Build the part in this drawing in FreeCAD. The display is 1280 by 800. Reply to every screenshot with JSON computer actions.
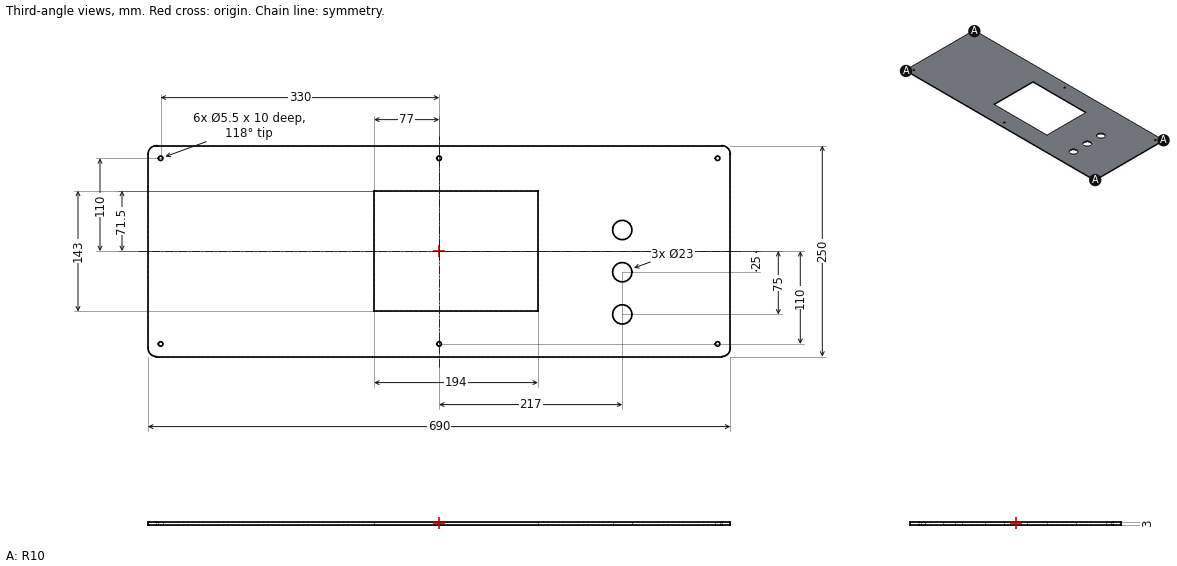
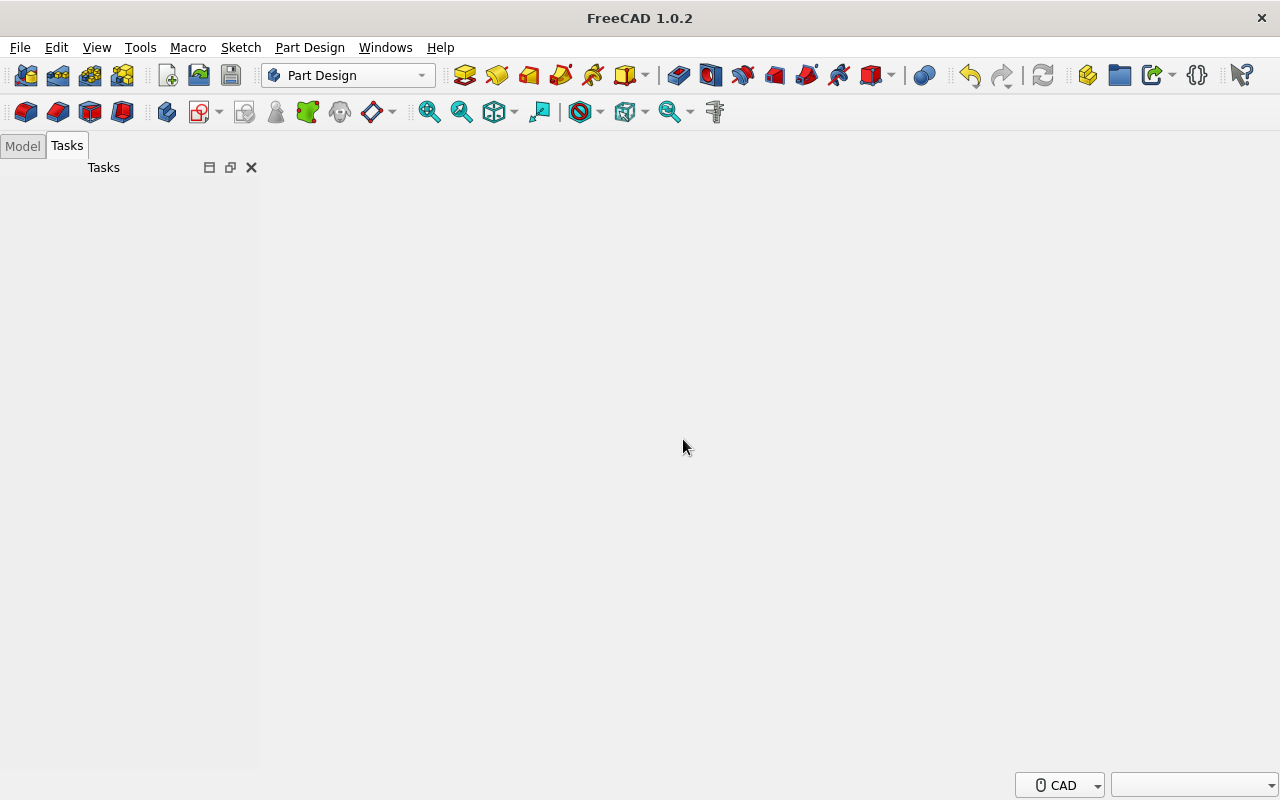
{"action": "left_click", "coordinate": [168, 76]}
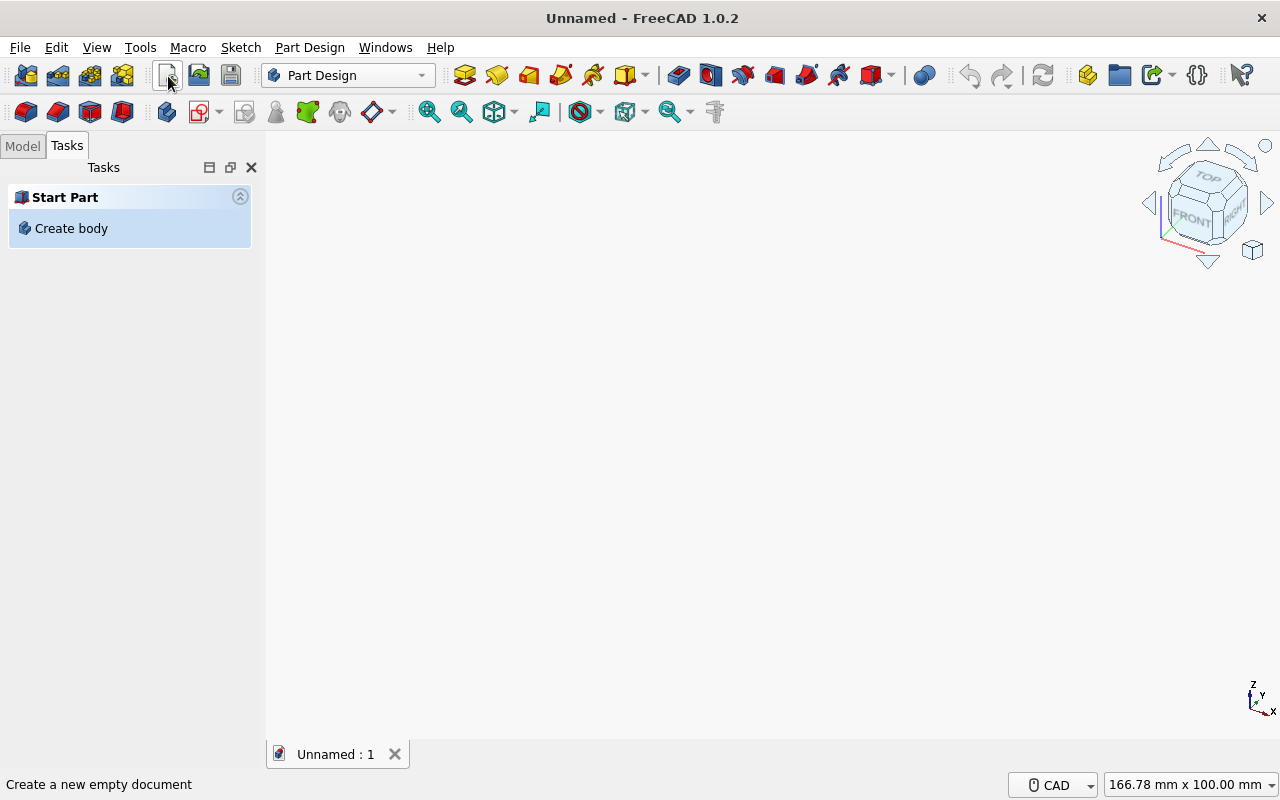
{"action": "left_click", "coordinate": [200, 112]}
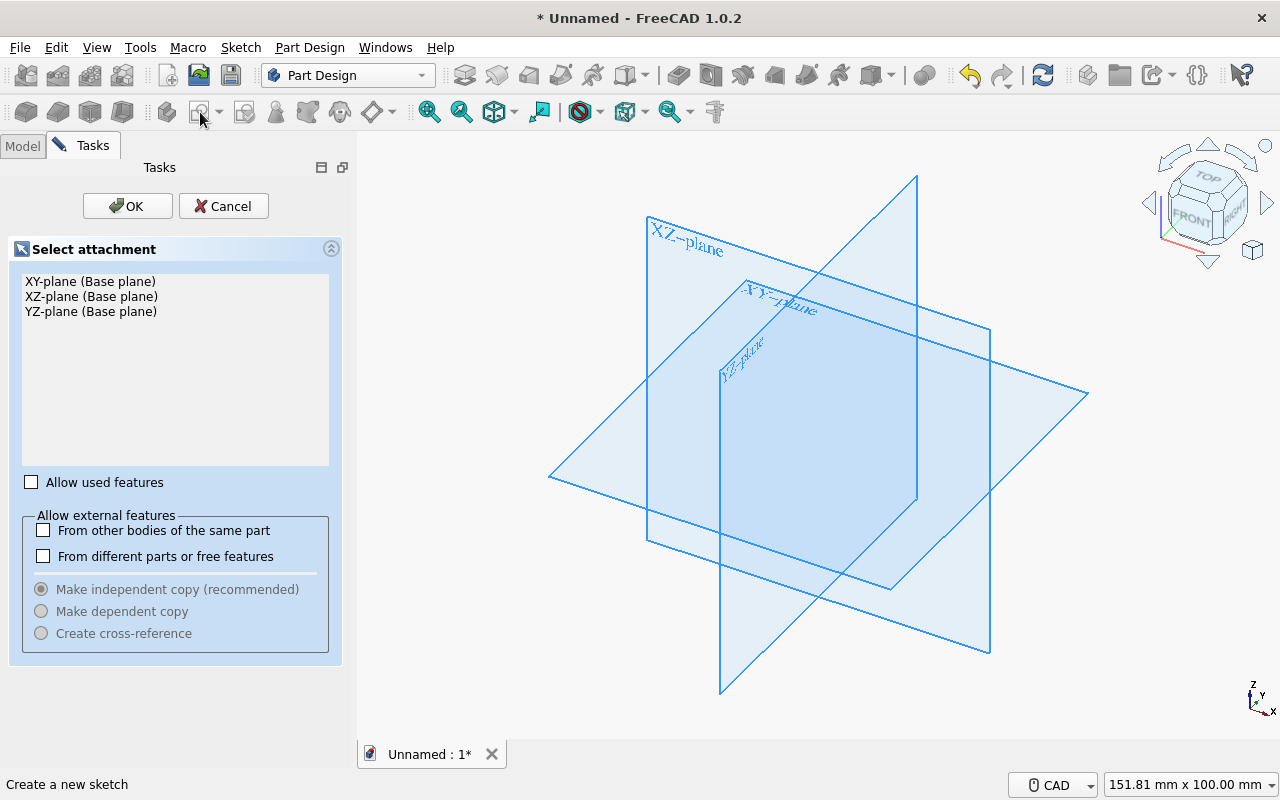
{"action": "left_click", "coordinate": [82, 282]}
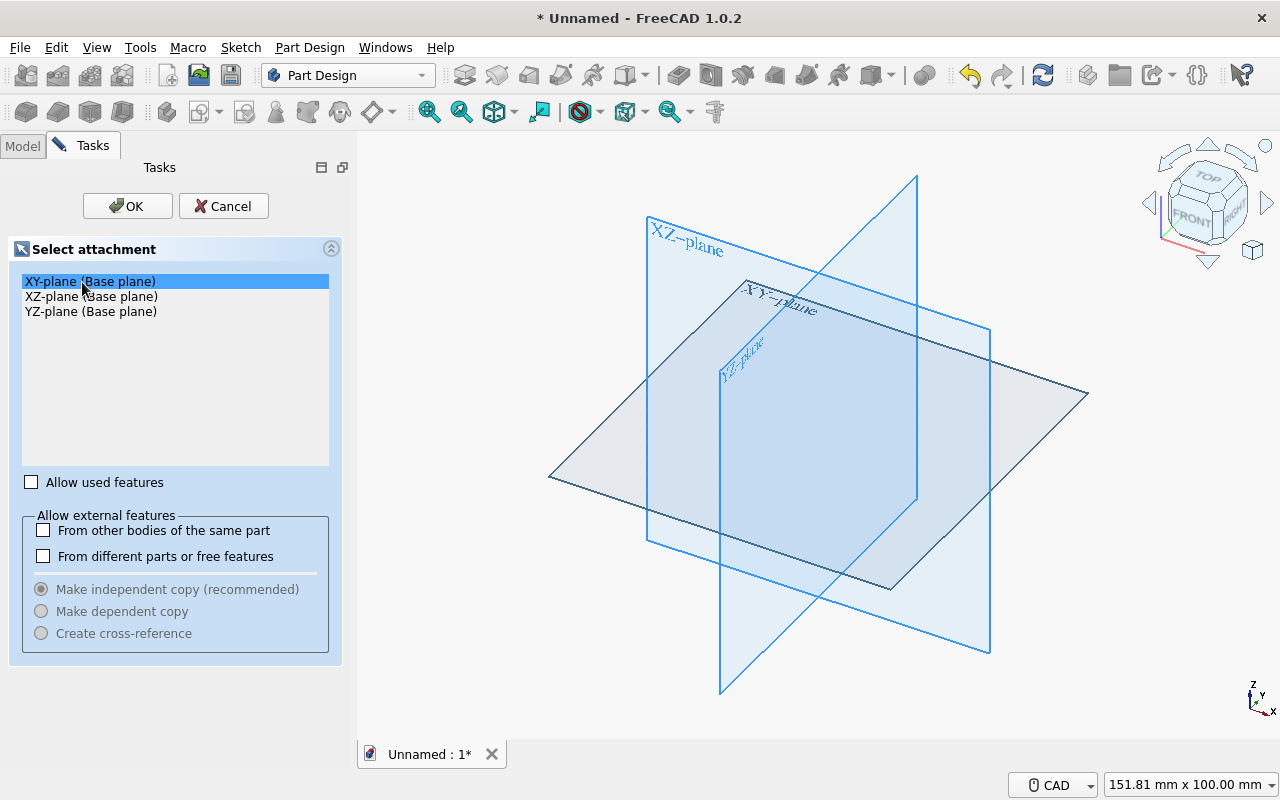
{"action": "left_click", "coordinate": [128, 206]}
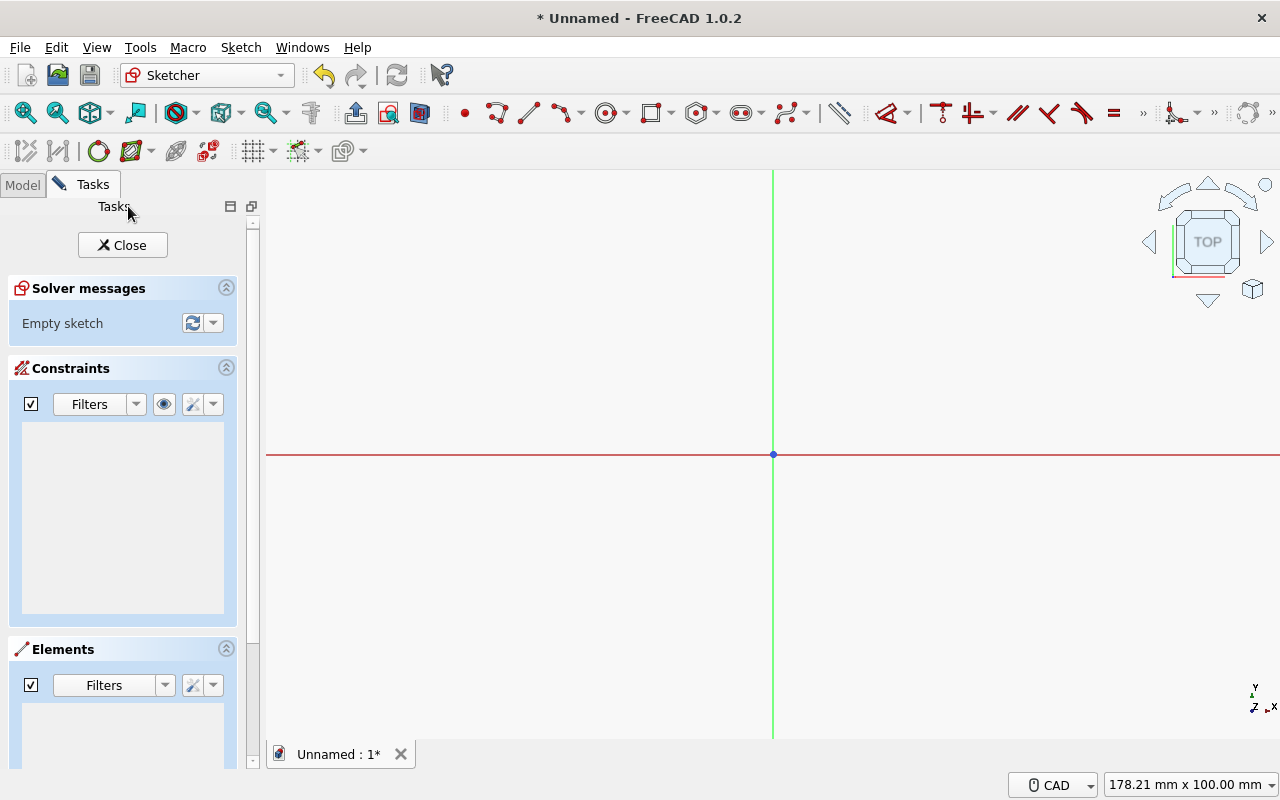
{"action": "scroll", "coordinate": [694, 454], "scroll_direction": "down", "scroll_amount": 10}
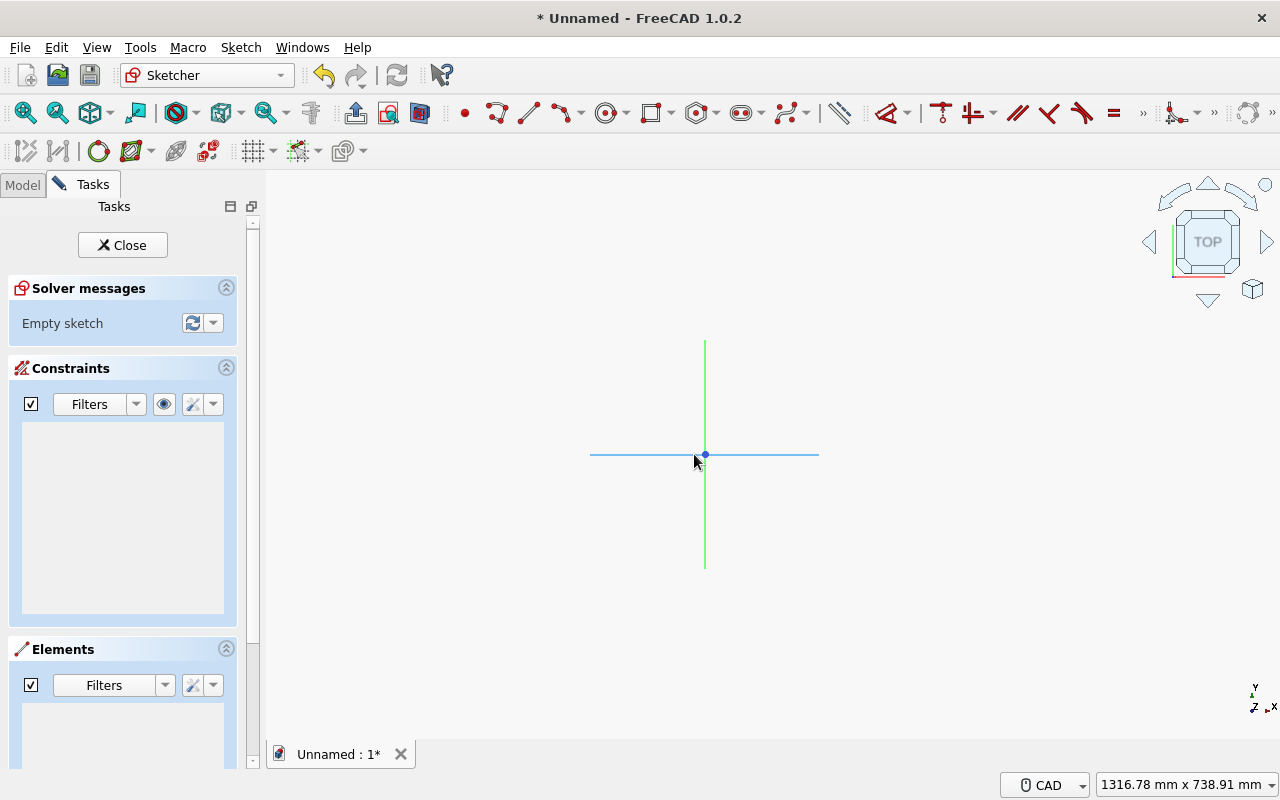
{"action": "key", "text": "g v"}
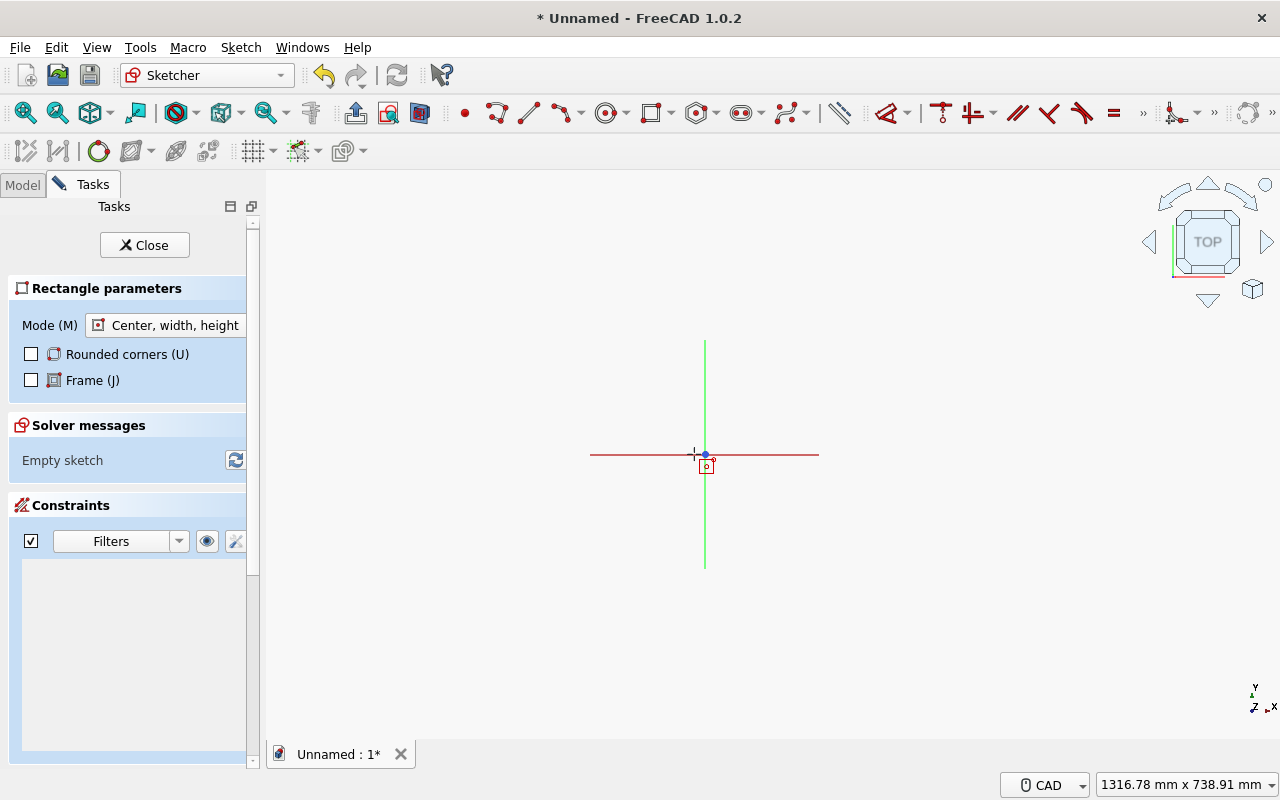
{"action": "left_click", "coordinate": [705, 454]}
{"action": "left_click", "coordinate": [971, 358]}
{"action": "key", "text": "Escape"}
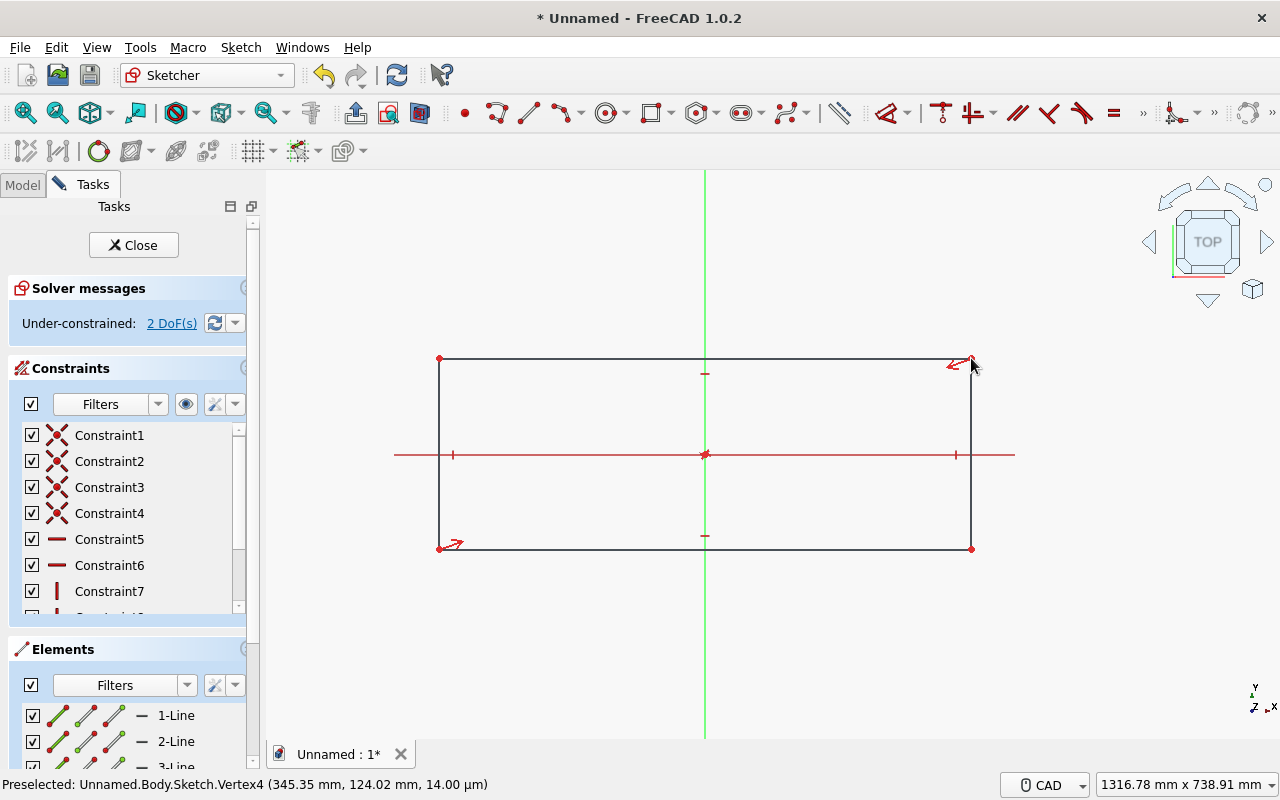
{"action": "left_click", "coordinate": [599, 550]}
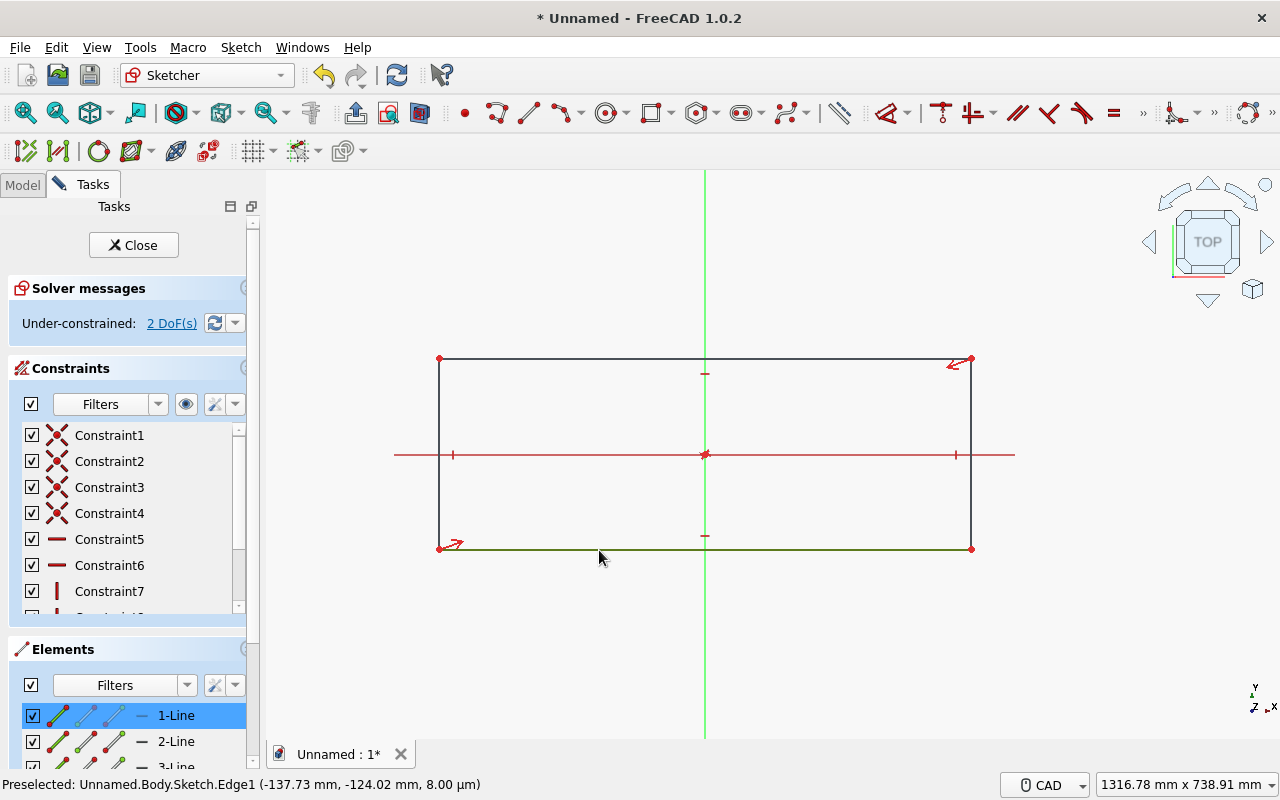
{"action": "left_click", "coordinate": [910, 114]}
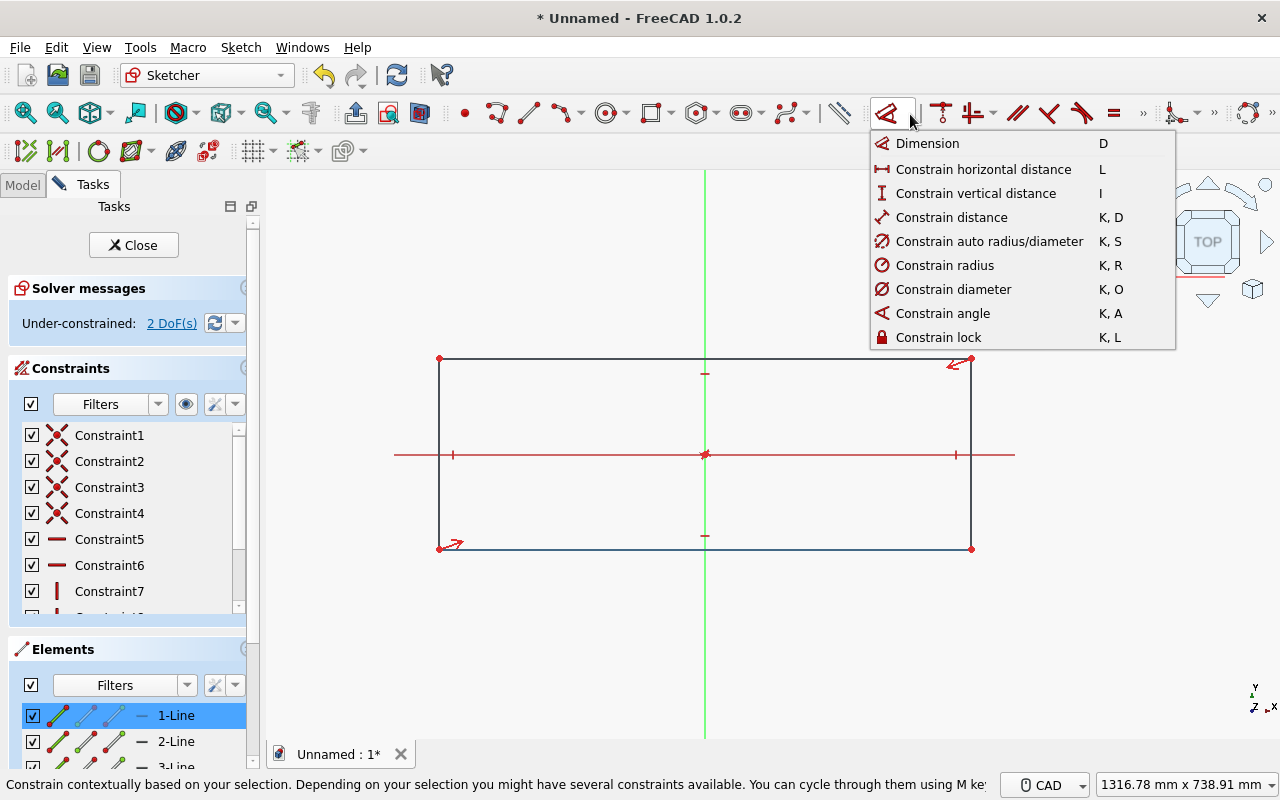
{"action": "left_click", "coordinate": [1023, 169]}